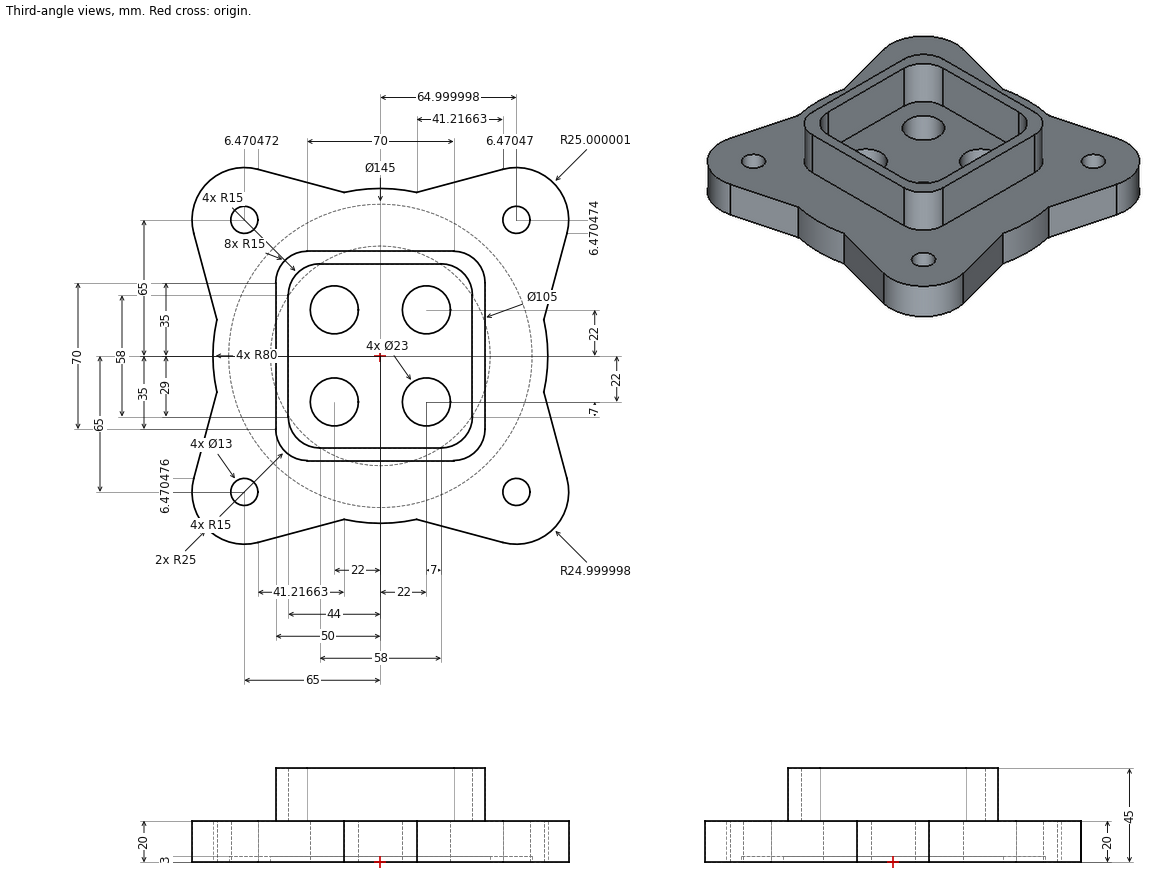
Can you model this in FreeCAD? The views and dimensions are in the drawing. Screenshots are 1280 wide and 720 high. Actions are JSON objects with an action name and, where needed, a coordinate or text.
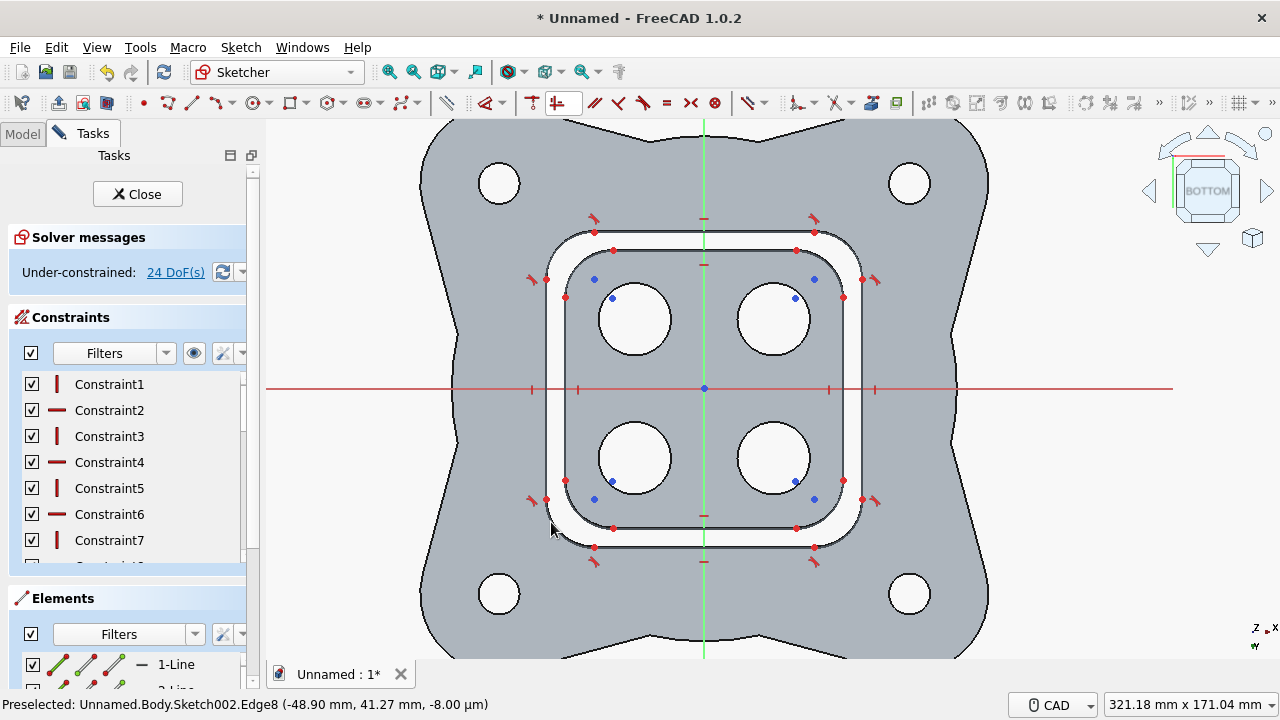
{"action": "left_click", "coordinate": [565, 353]}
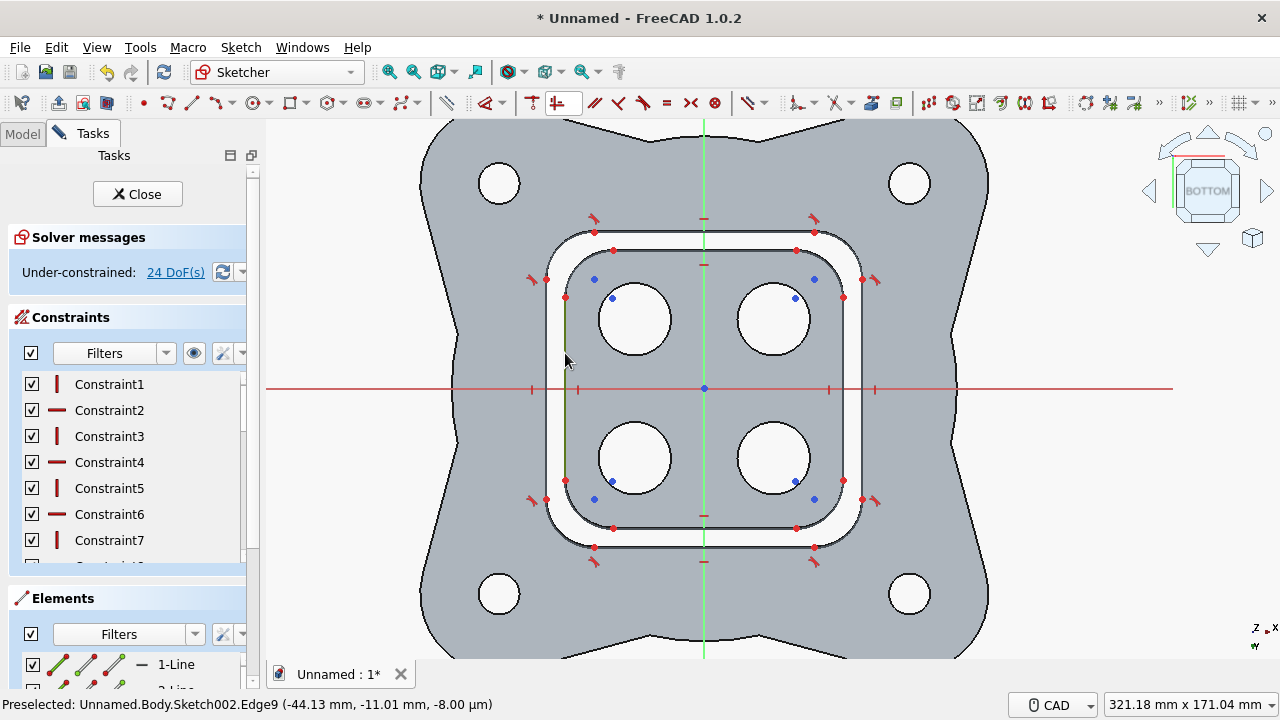
{"action": "left_click", "coordinate": [570, 503]}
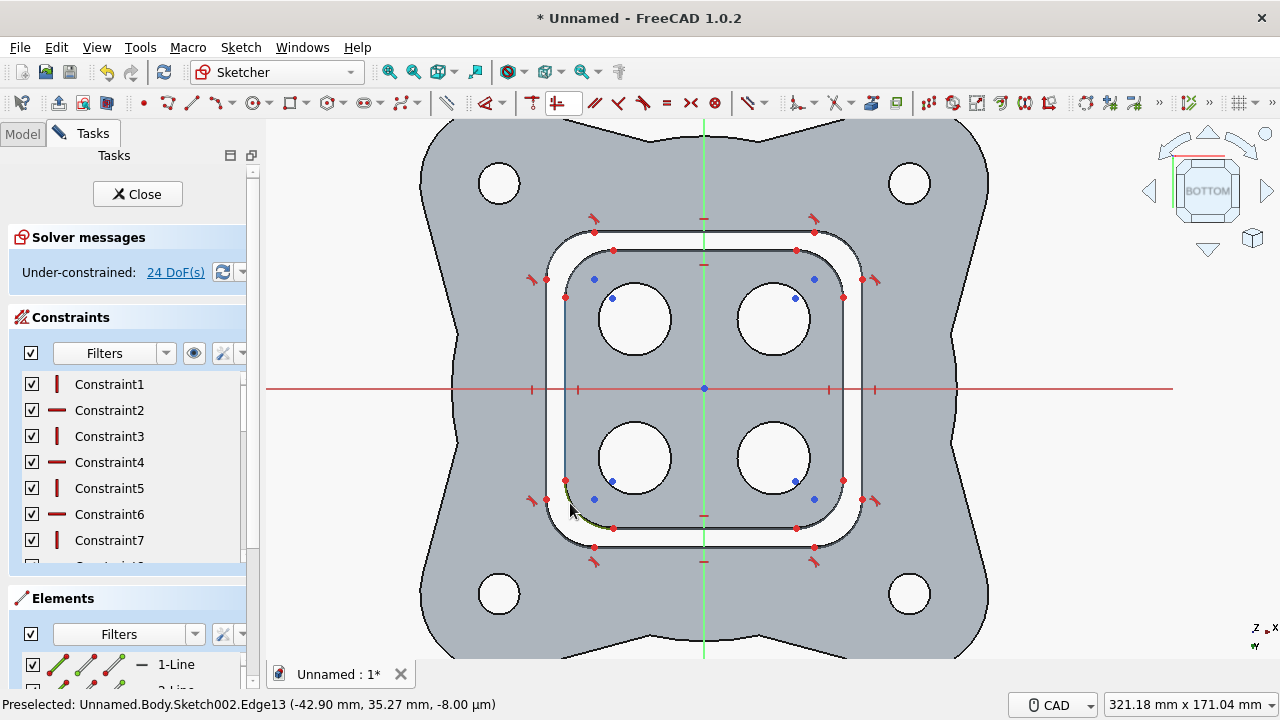
{"action": "left_click", "coordinate": [644, 104]}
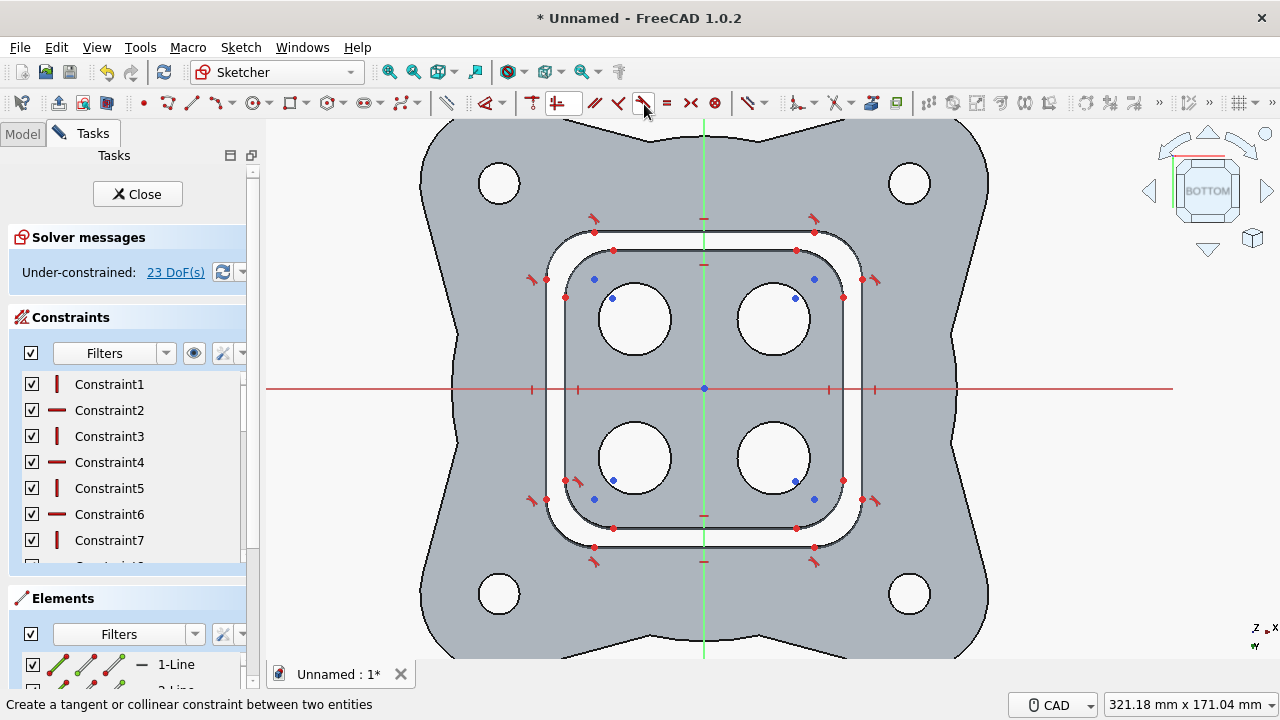
{"action": "left_click", "coordinate": [565, 353]}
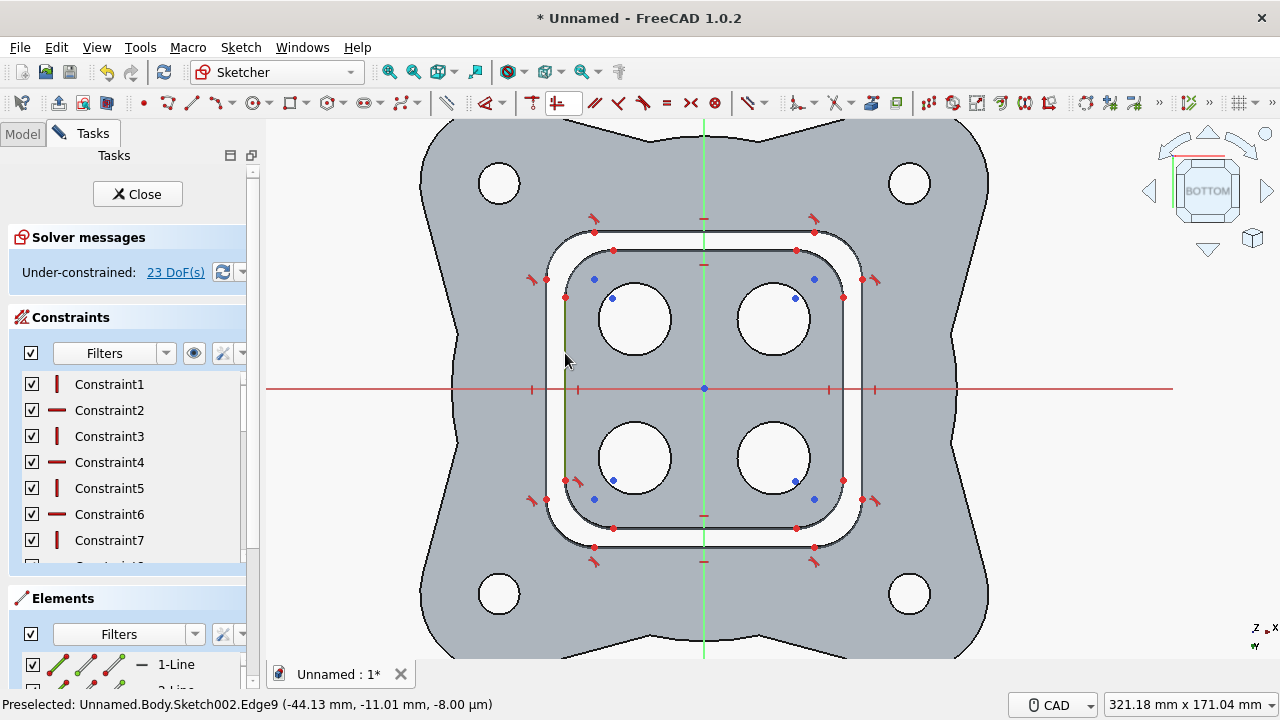
{"action": "left_click", "coordinate": [591, 256]}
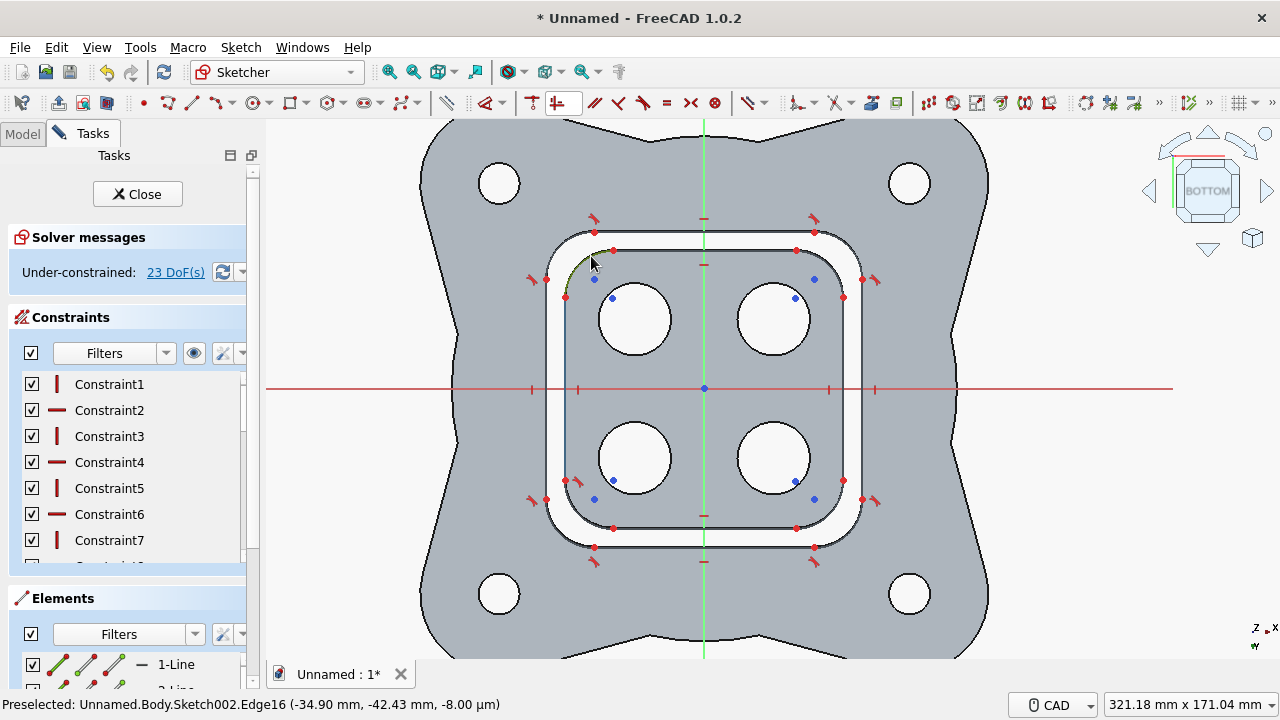
{"action": "left_click", "coordinate": [644, 104]}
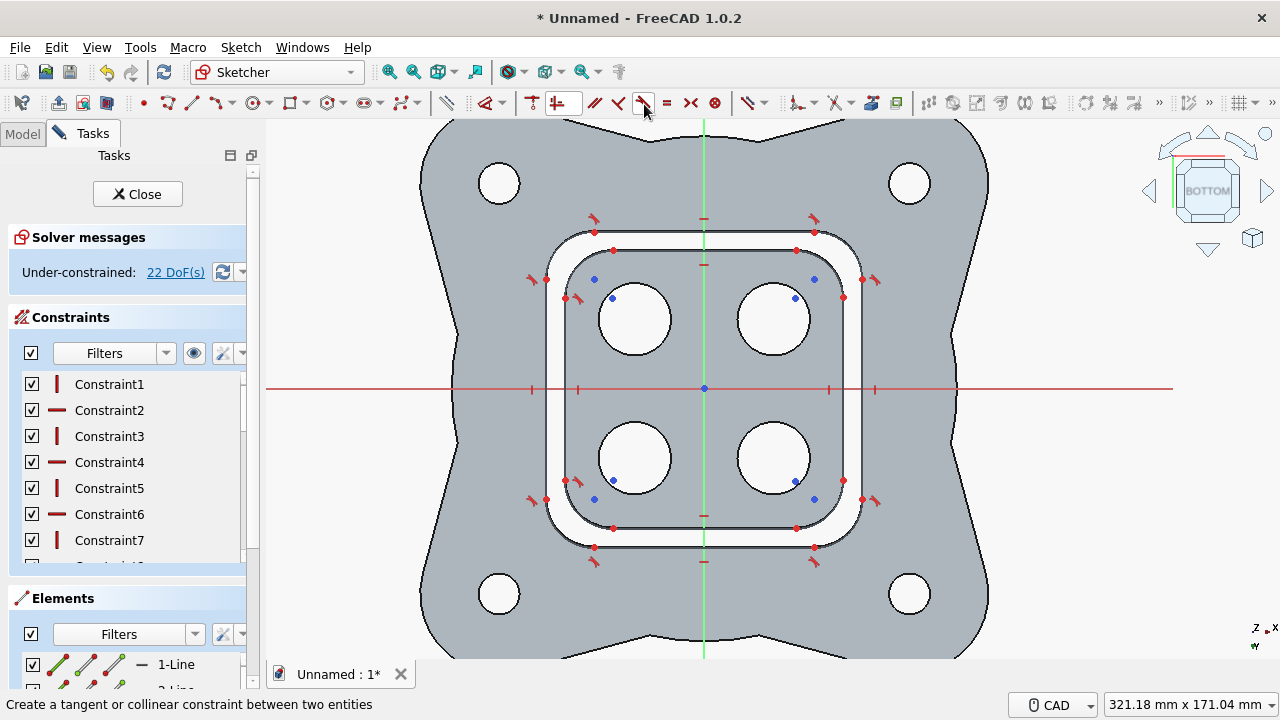
{"action": "left_click", "coordinate": [668, 529]}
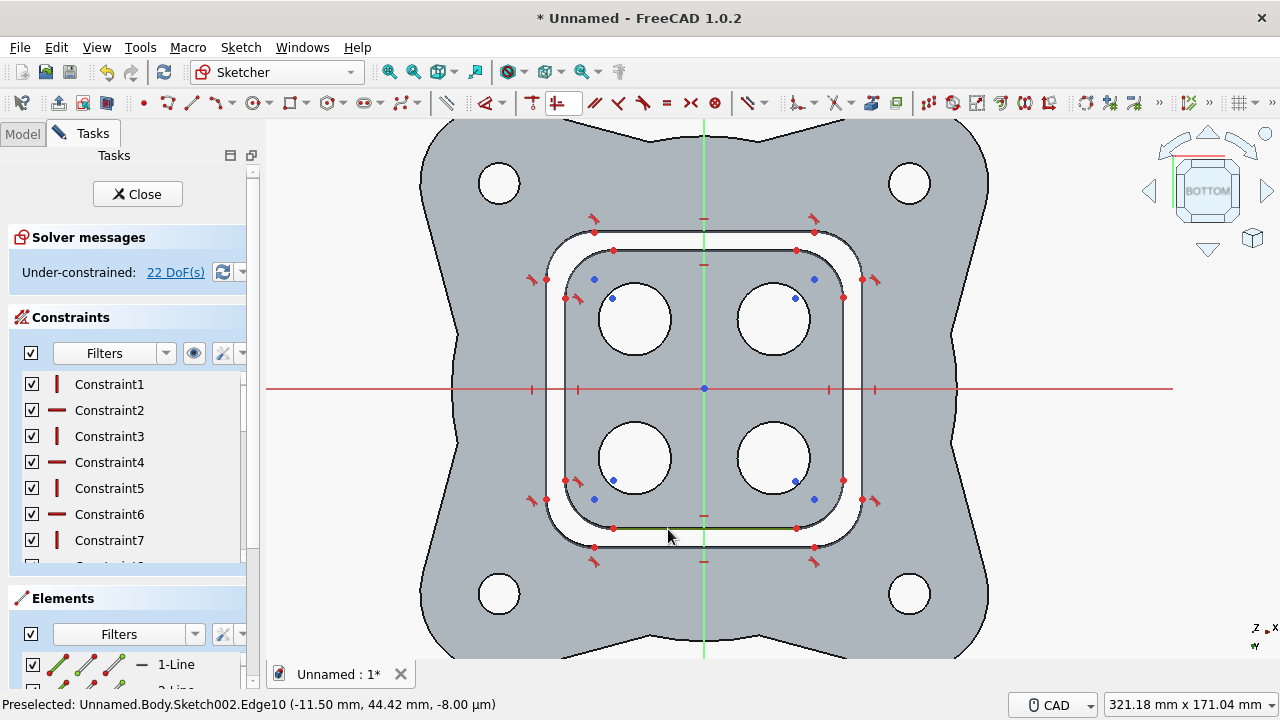
{"action": "left_click", "coordinate": [570, 503]}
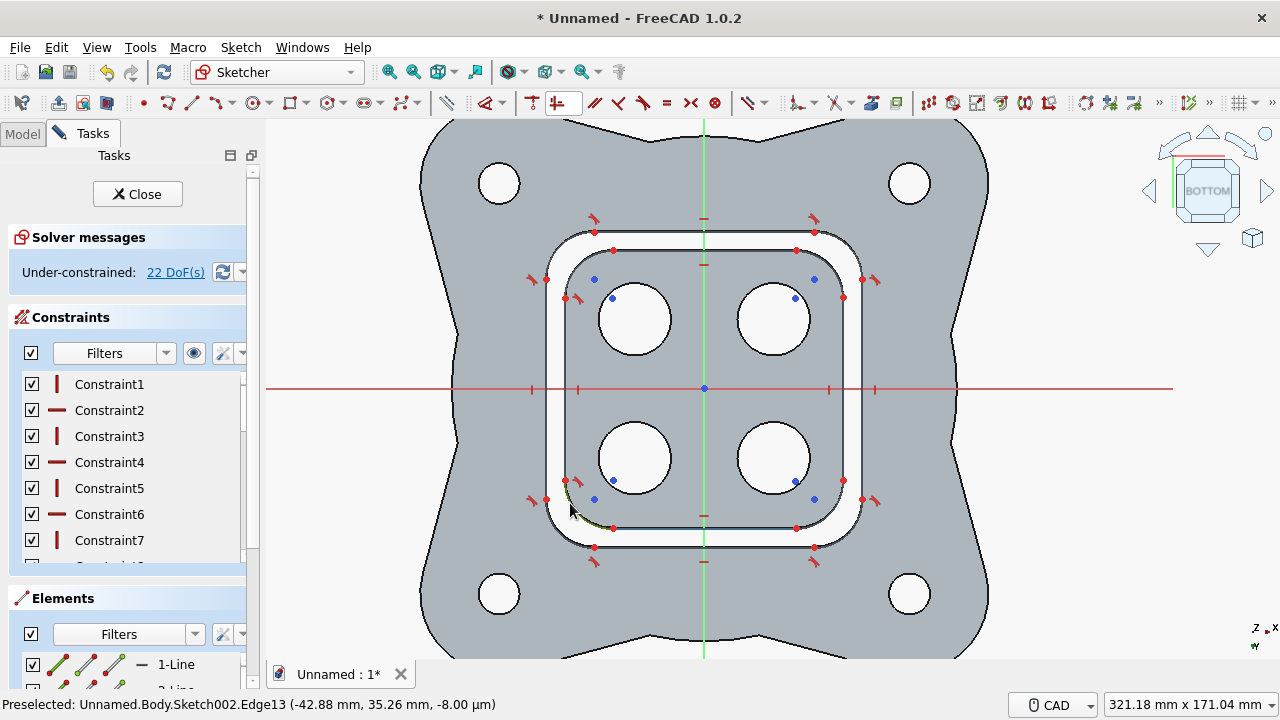
{"action": "left_click", "coordinate": [644, 104]}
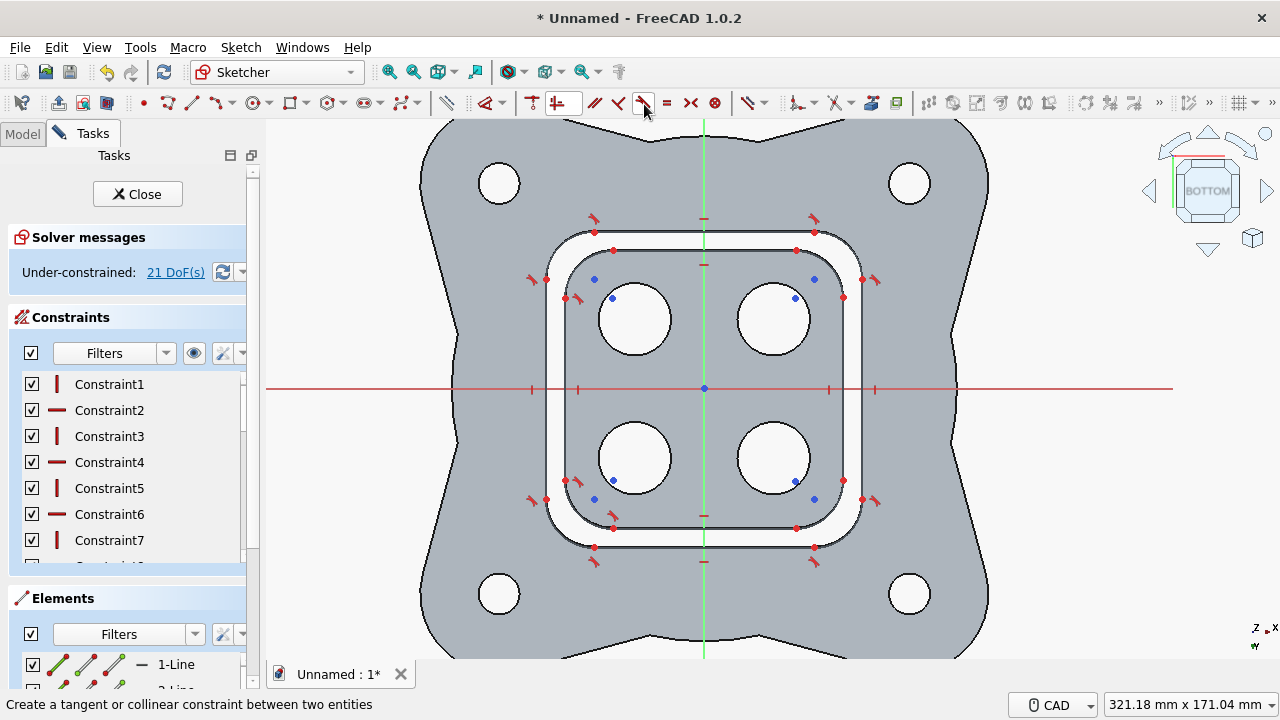
{"action": "left_click", "coordinate": [668, 529]}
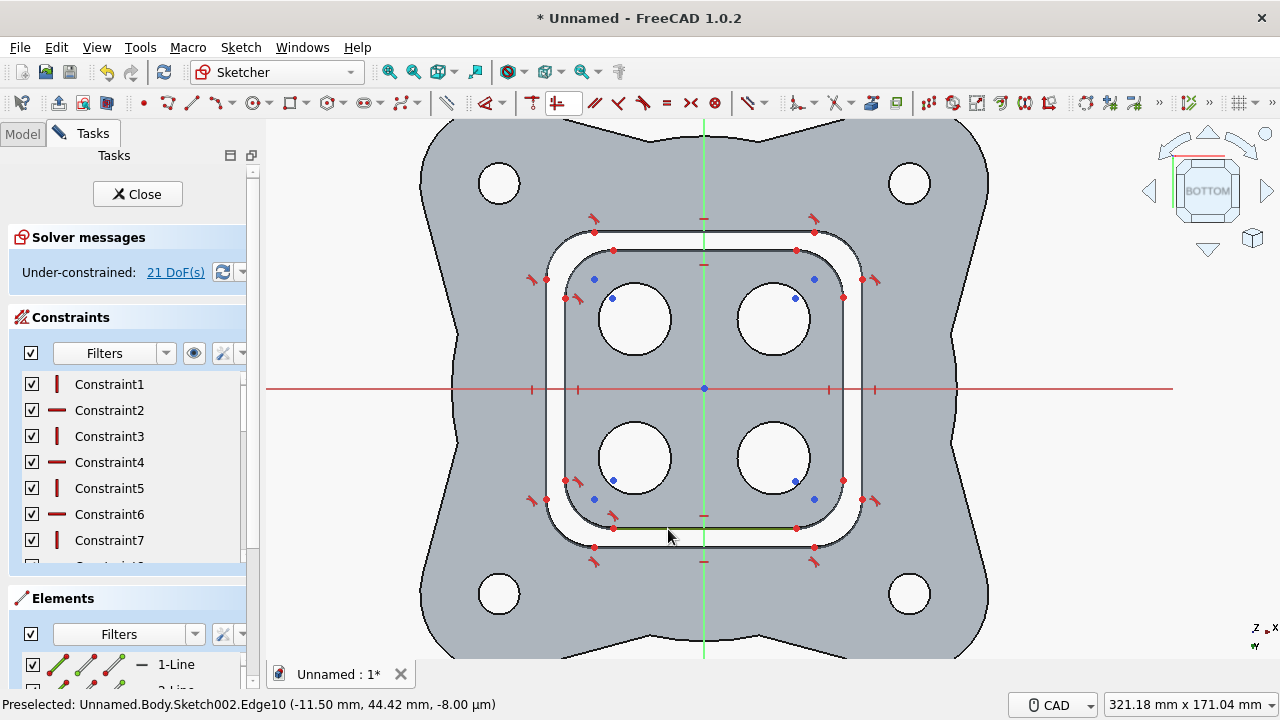
{"action": "left_click", "coordinate": [817, 524]}